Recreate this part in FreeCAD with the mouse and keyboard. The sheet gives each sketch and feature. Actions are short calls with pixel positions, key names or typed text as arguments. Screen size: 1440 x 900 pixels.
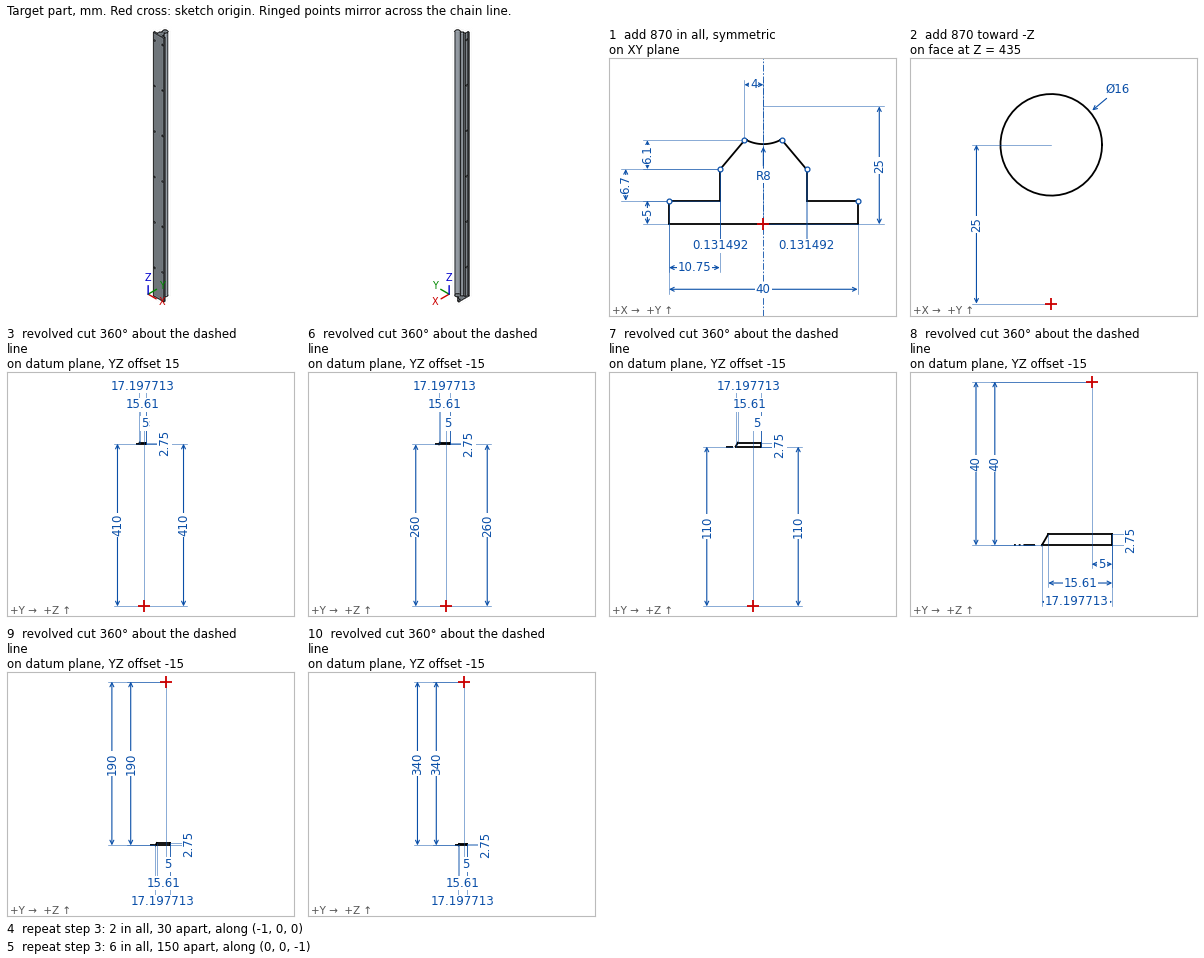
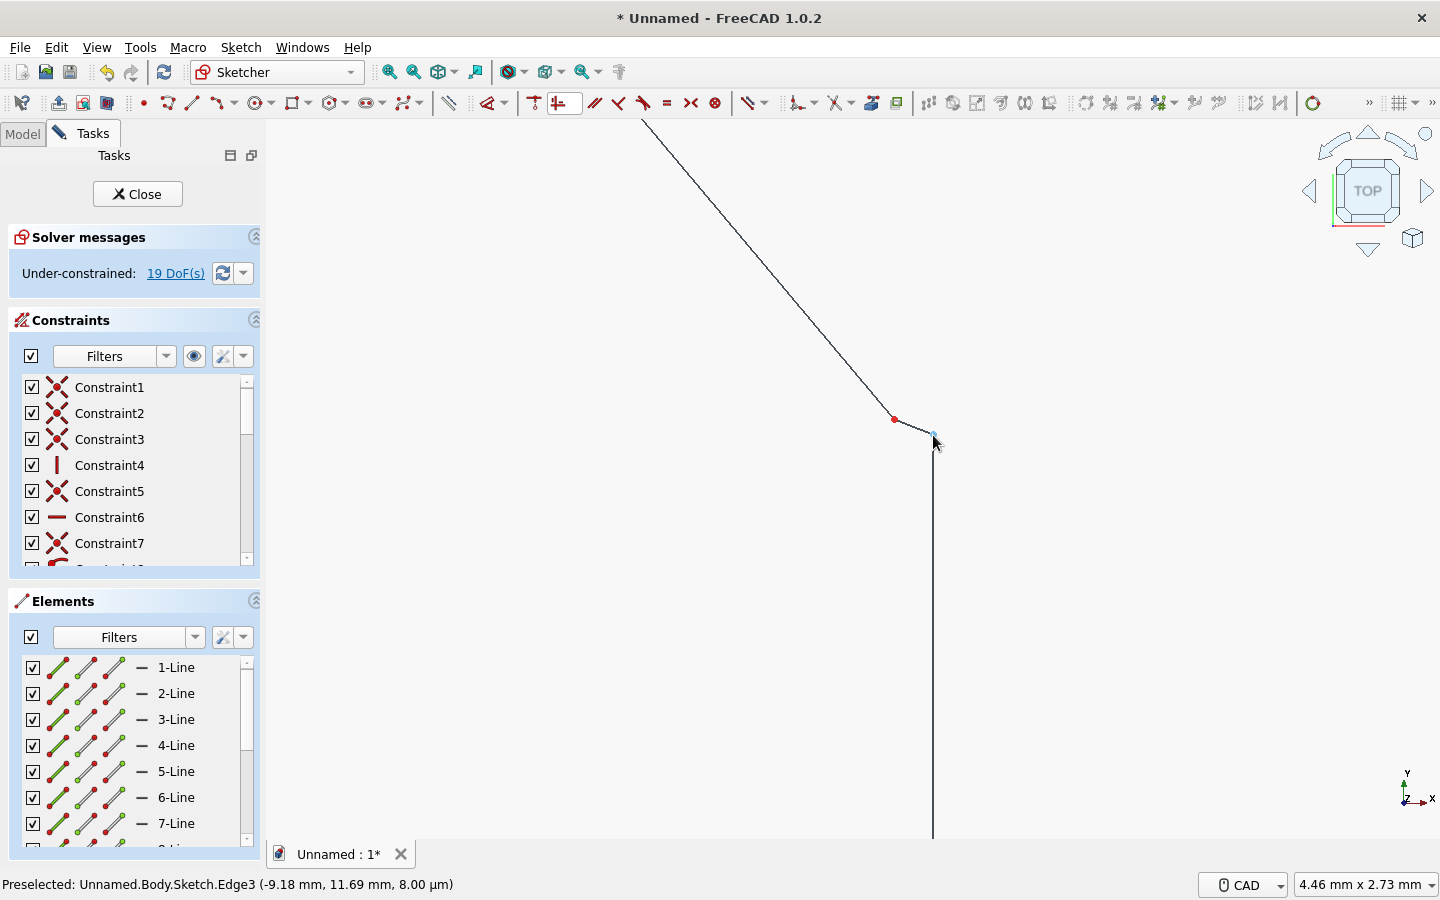
click(921, 430)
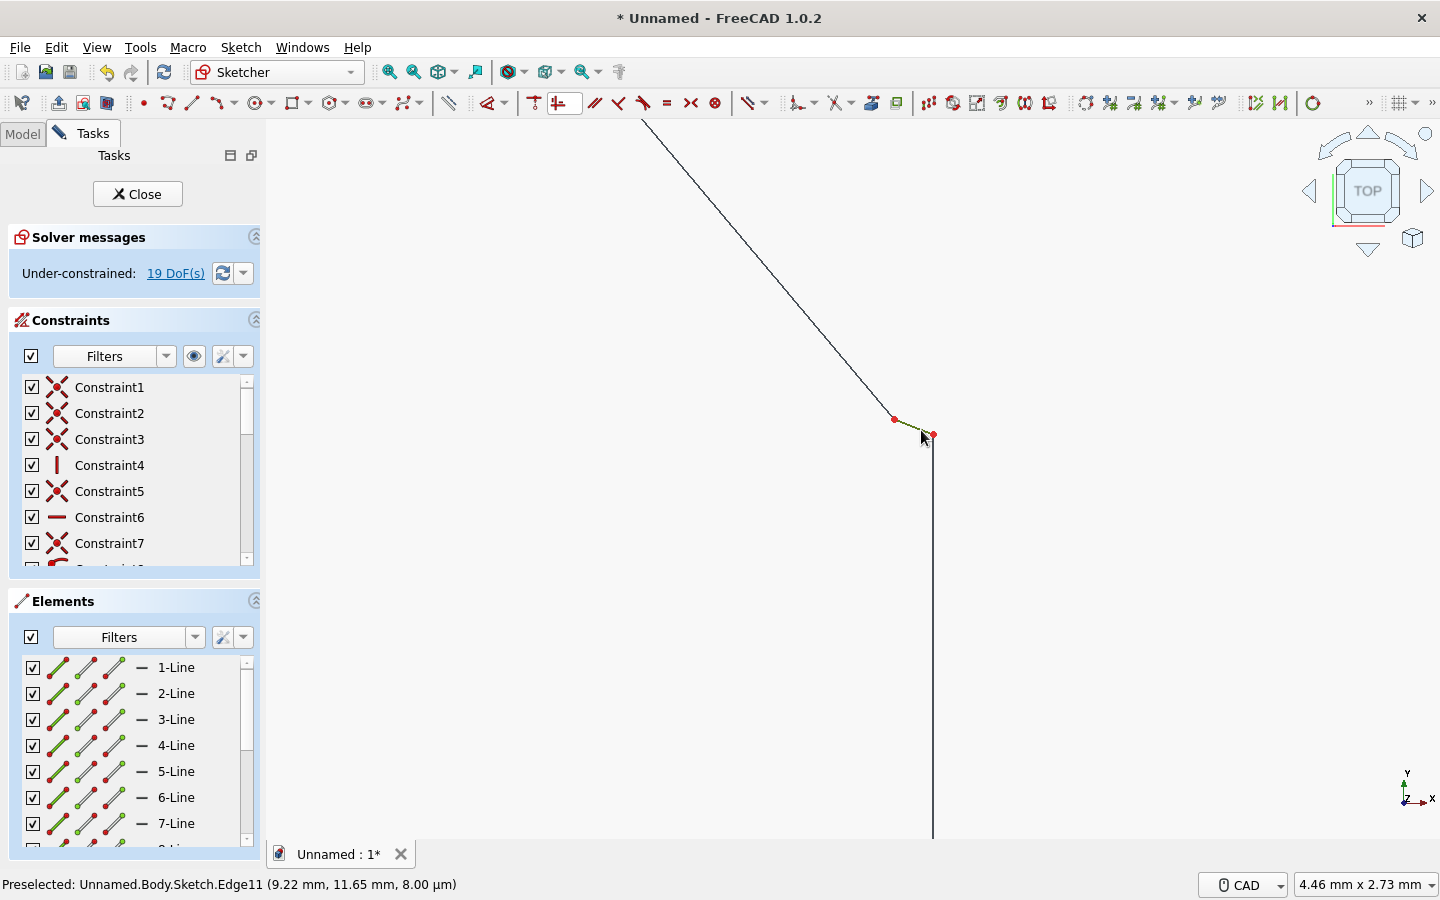
click(576, 104)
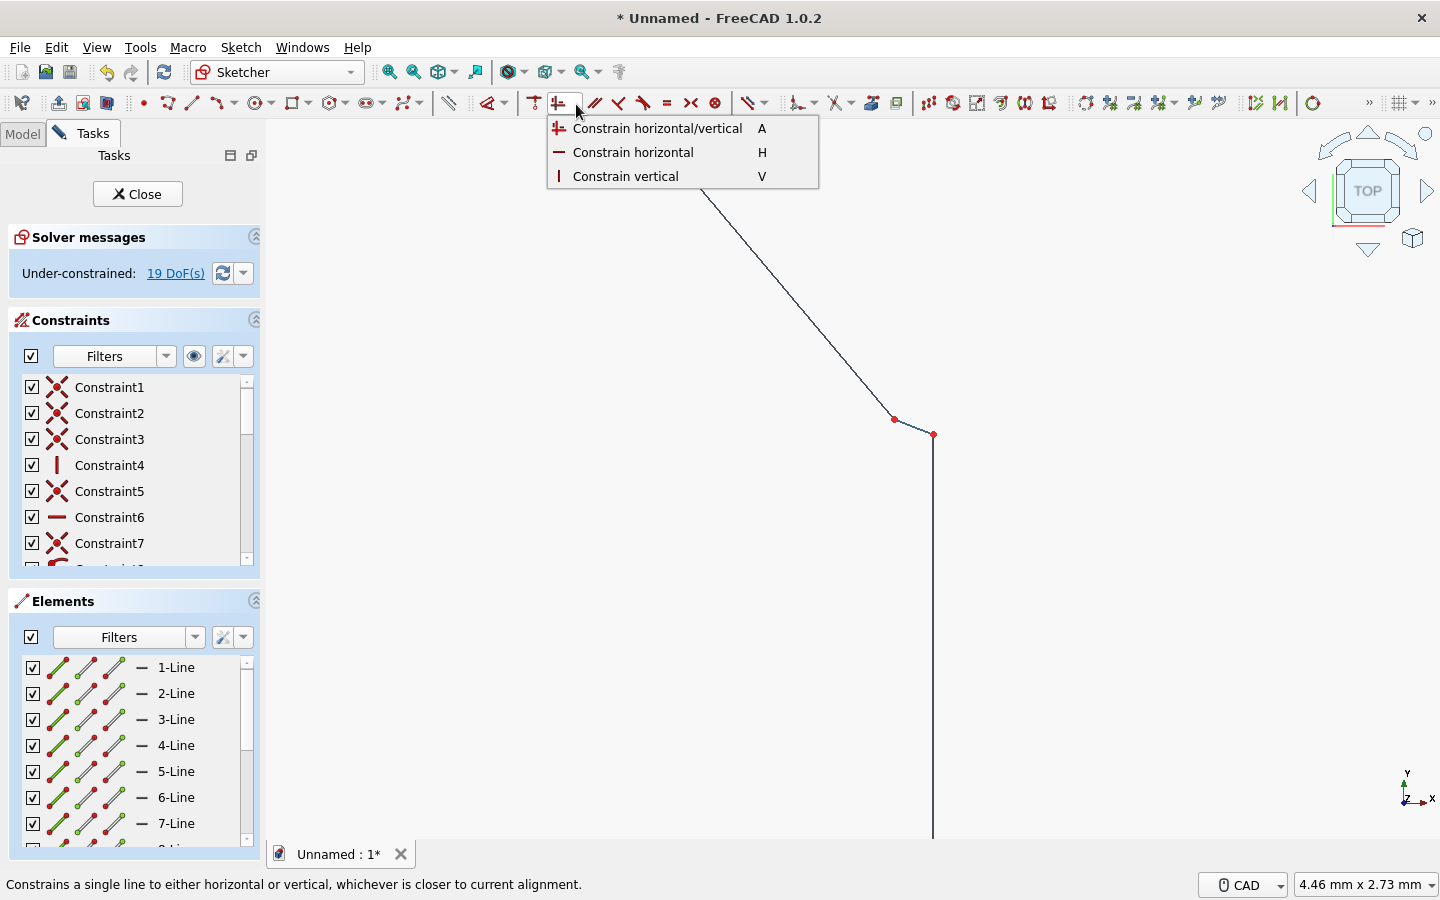
click(683, 152)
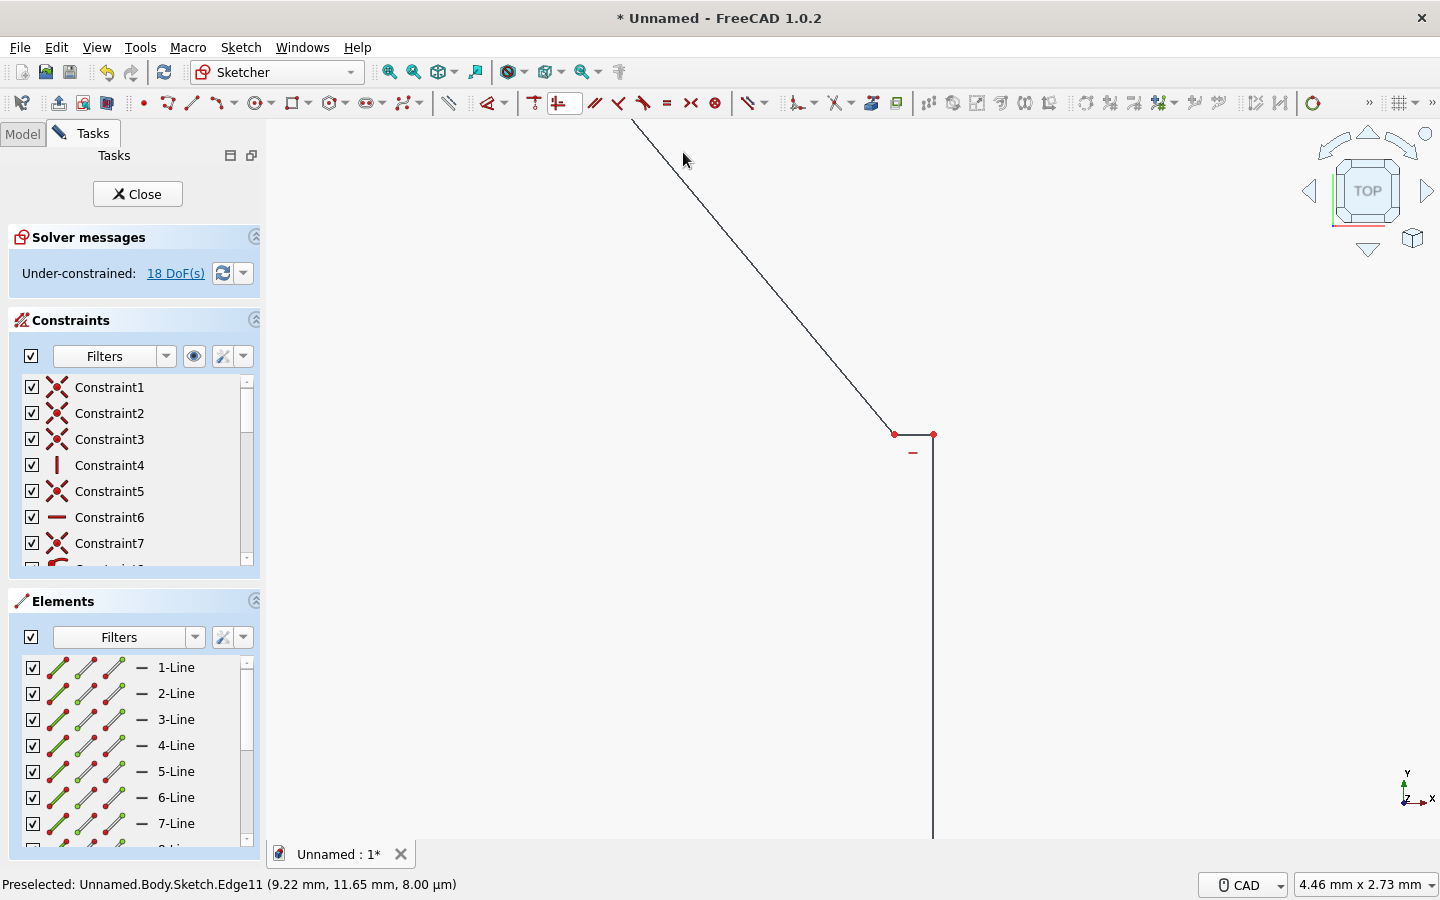
scroll(933, 435, down, 14)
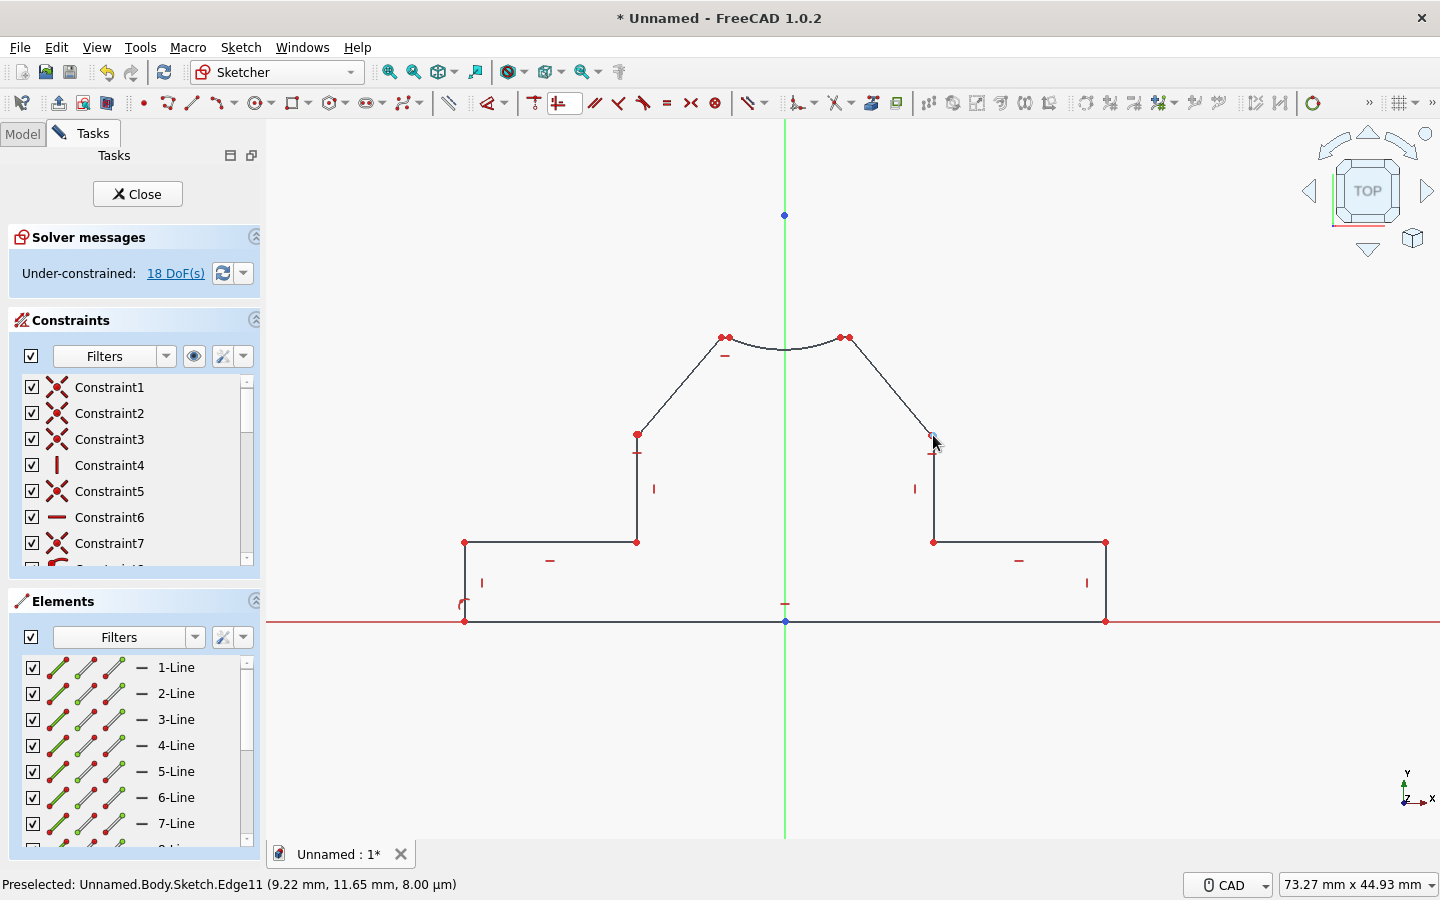
scroll(847, 337, up, 9)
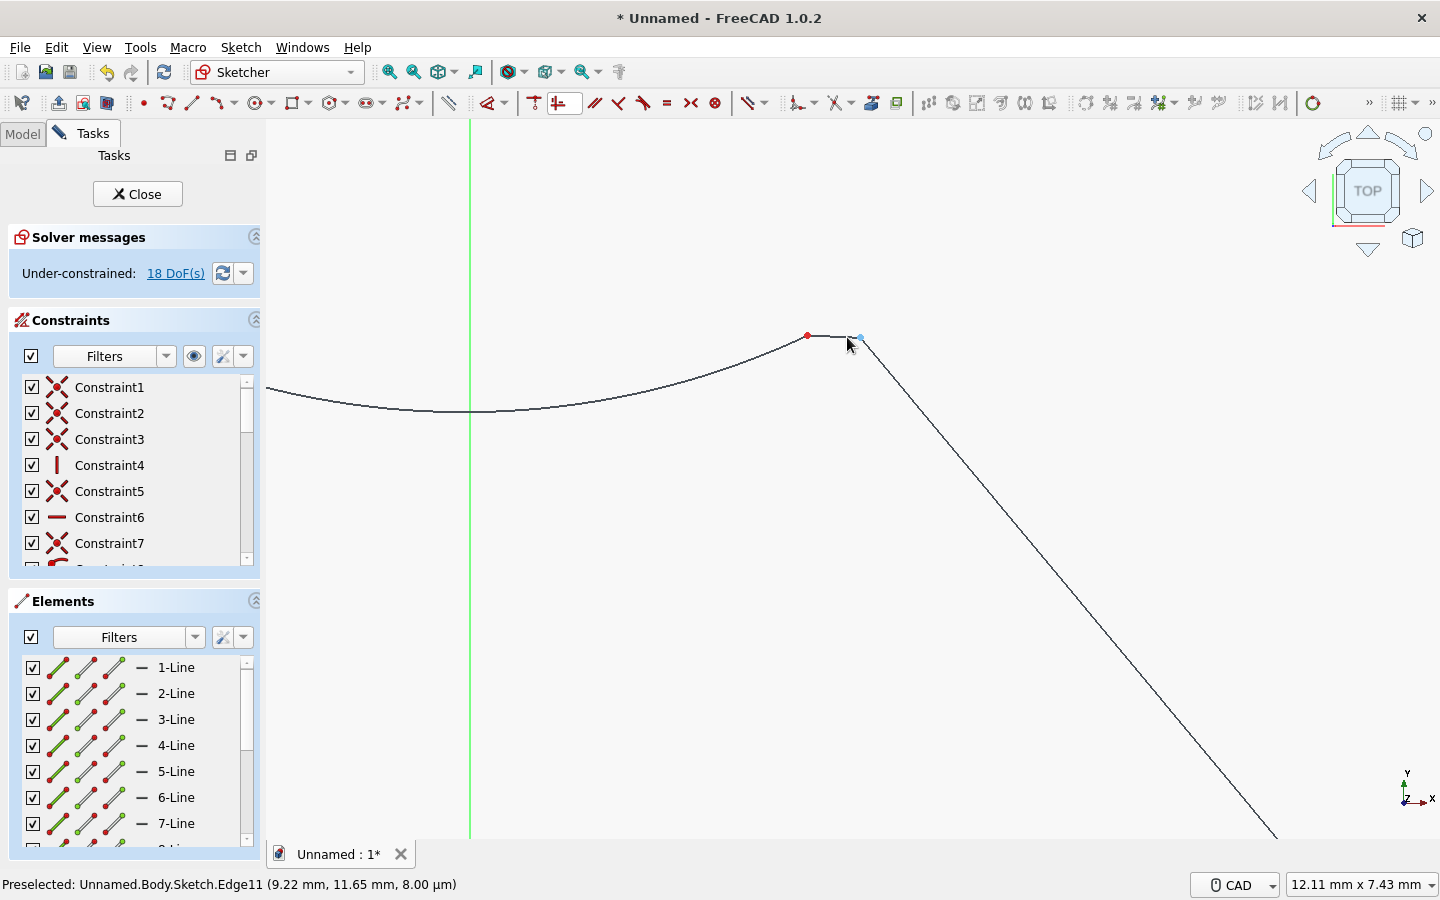
click(845, 337)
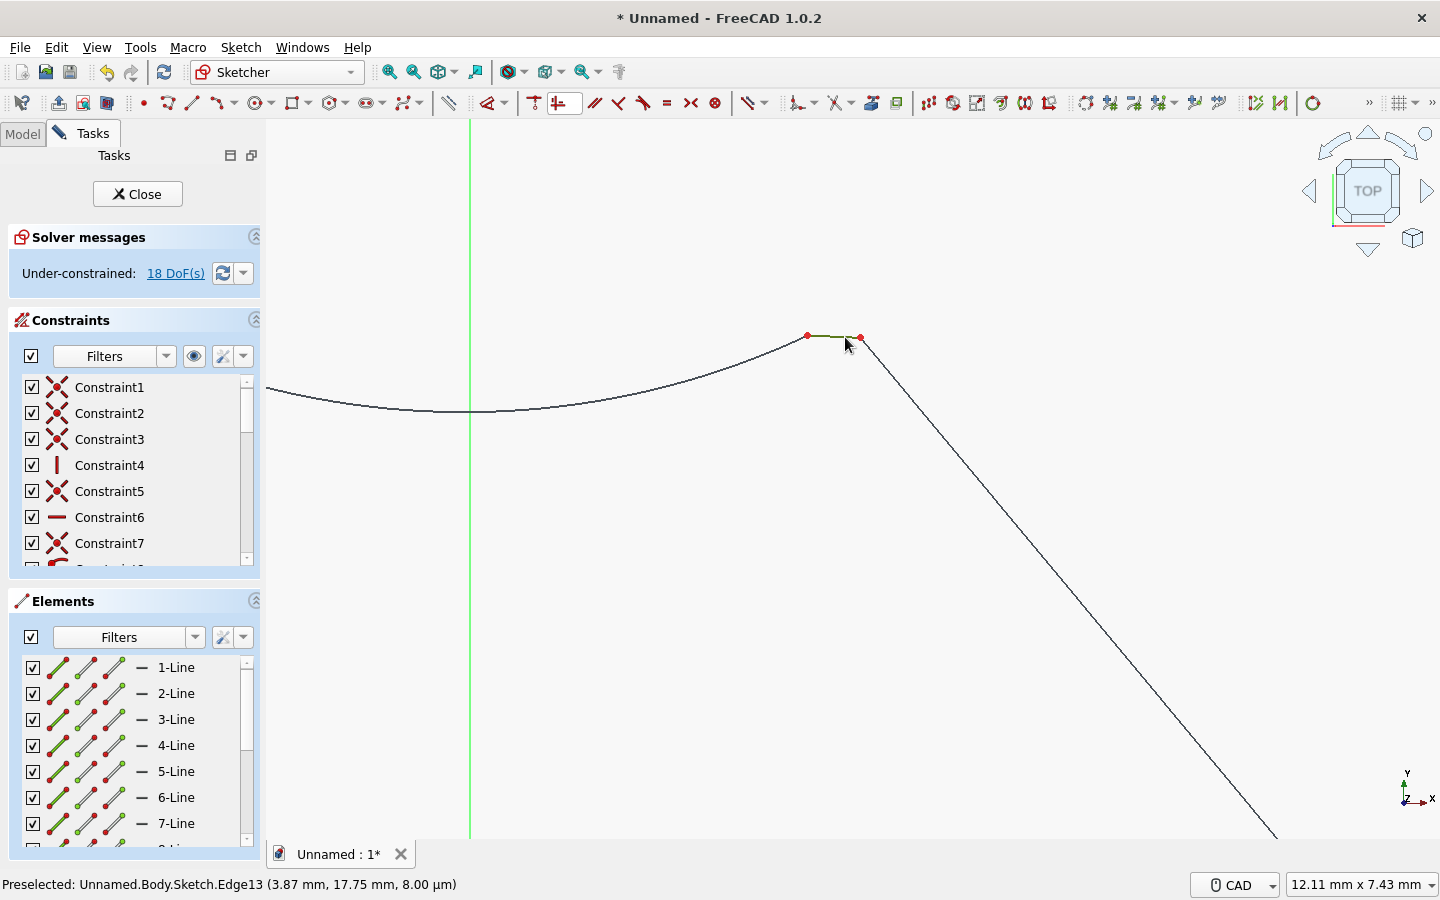
click(576, 104)